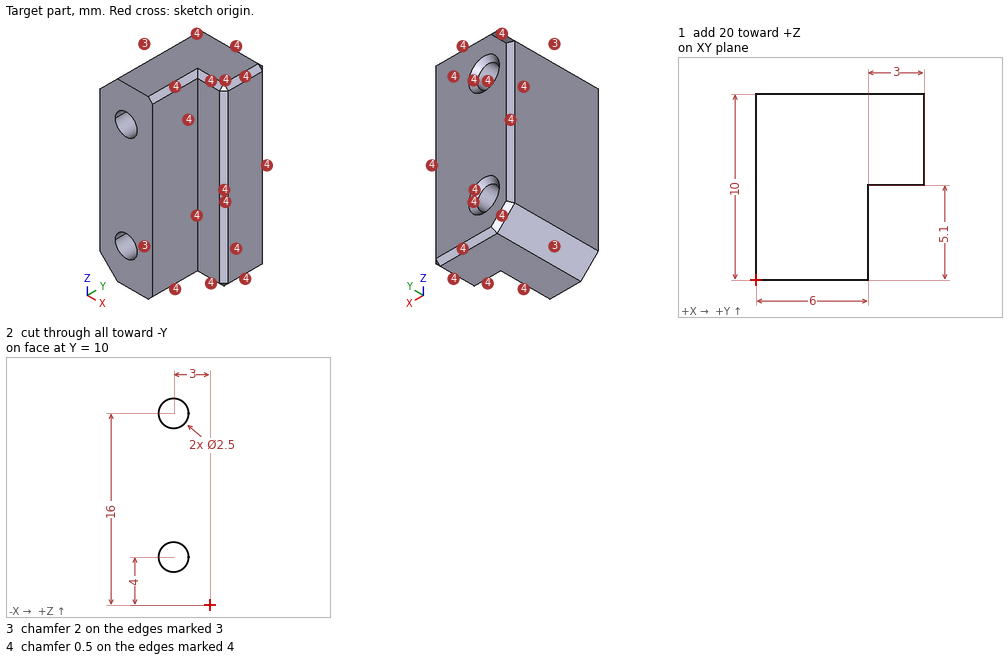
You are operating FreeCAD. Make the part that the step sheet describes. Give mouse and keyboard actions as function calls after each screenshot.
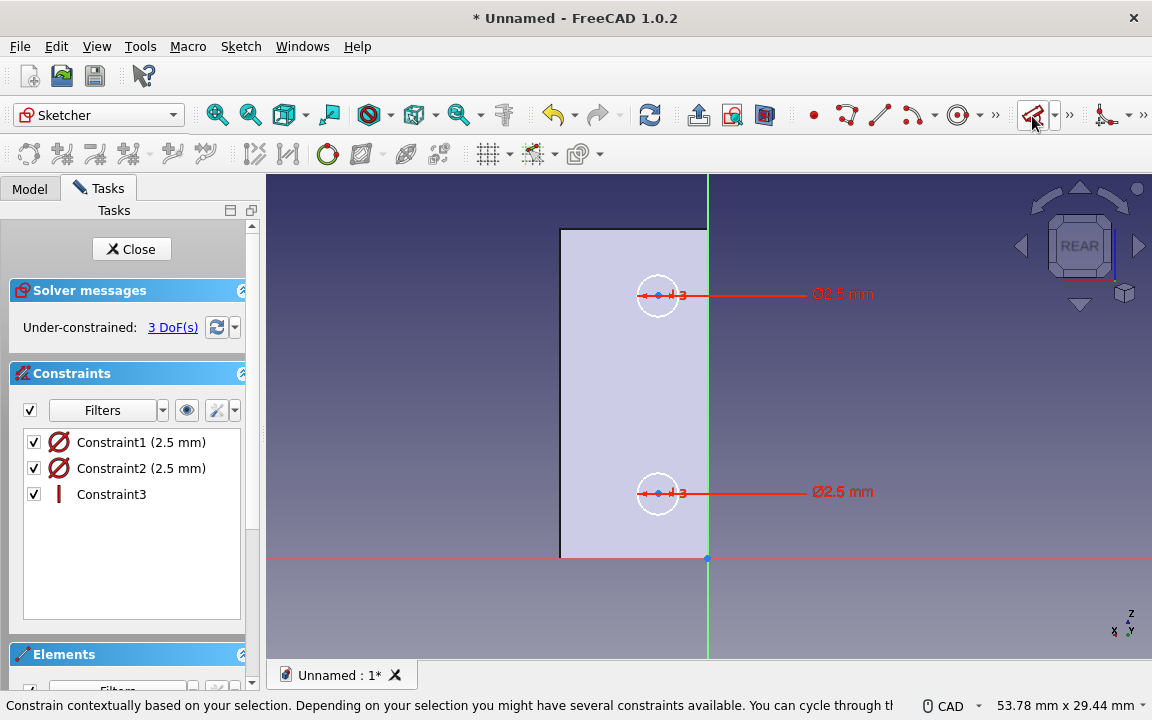
click(658, 296)
click(683, 593)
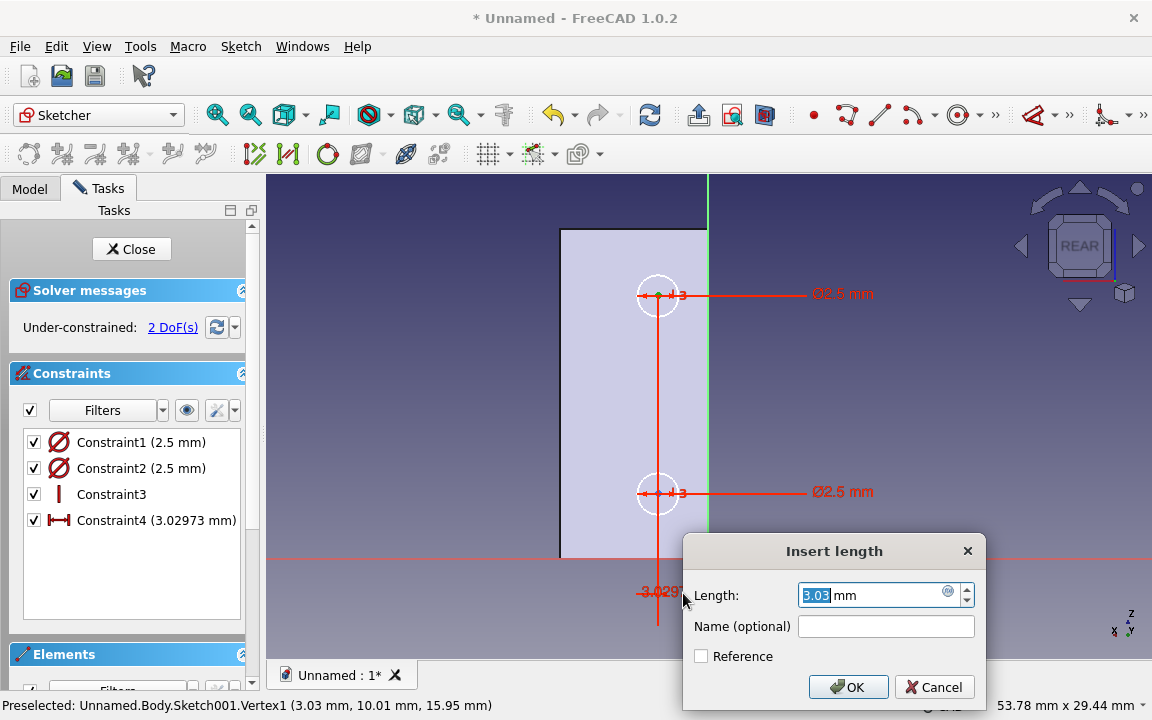
text(3)
key(Return)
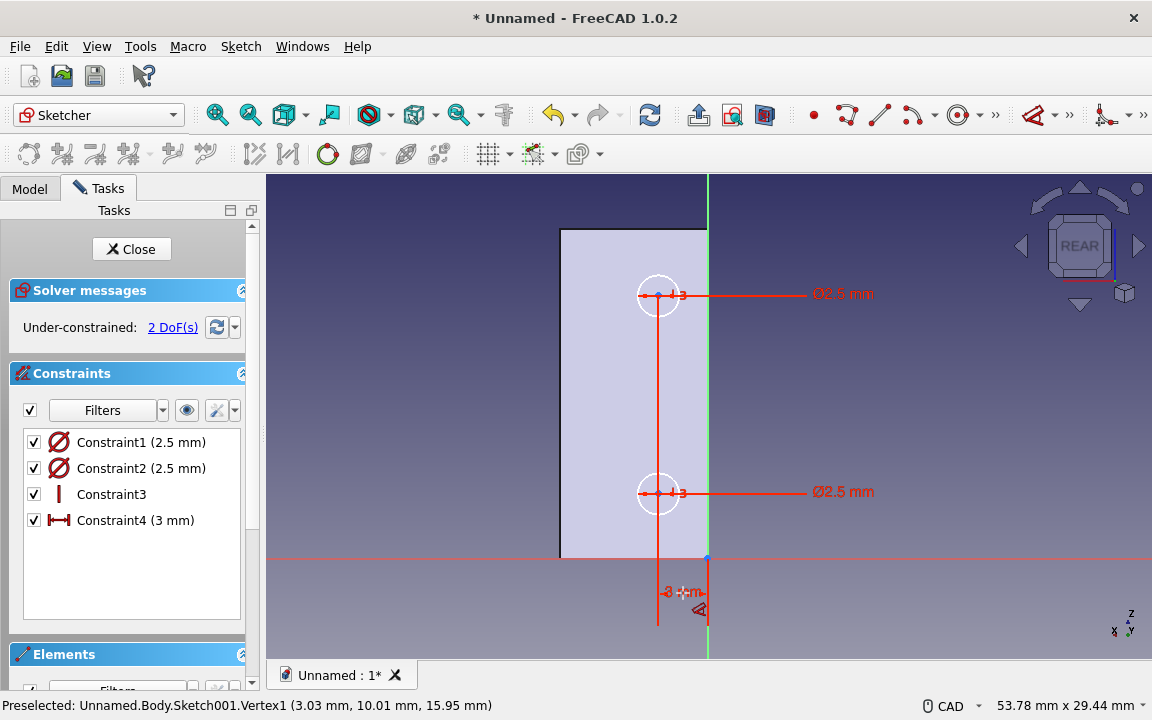
click(658, 494)
click(742, 526)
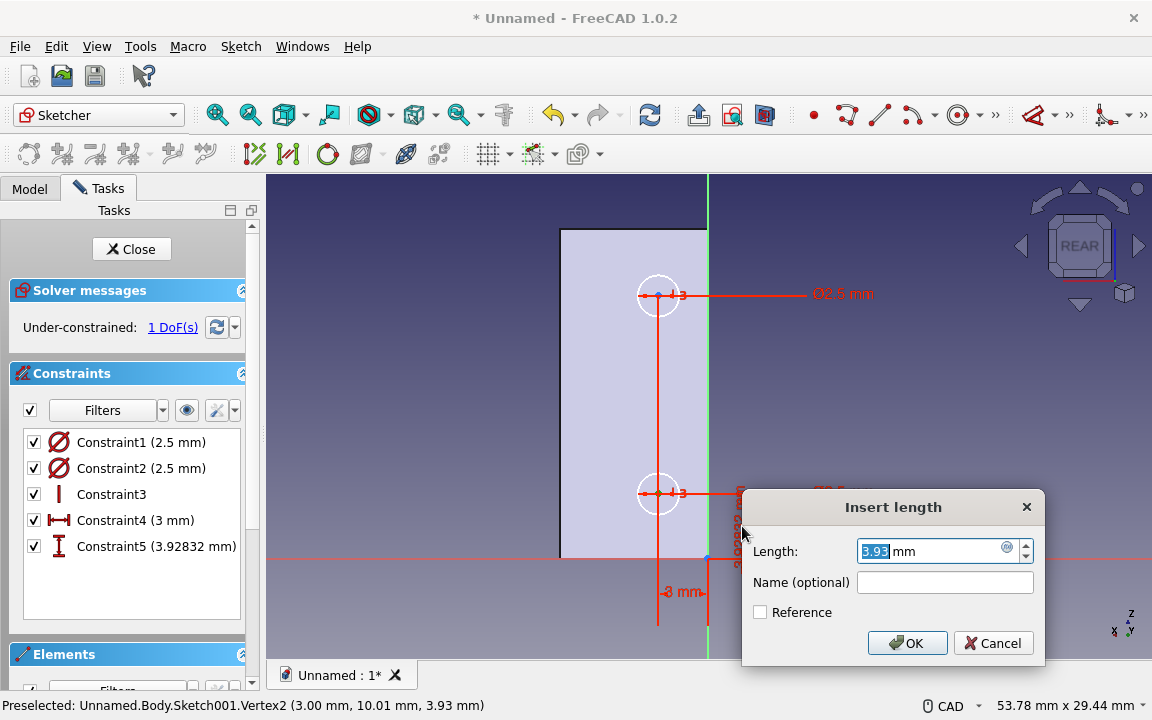
text(4)
key(Return)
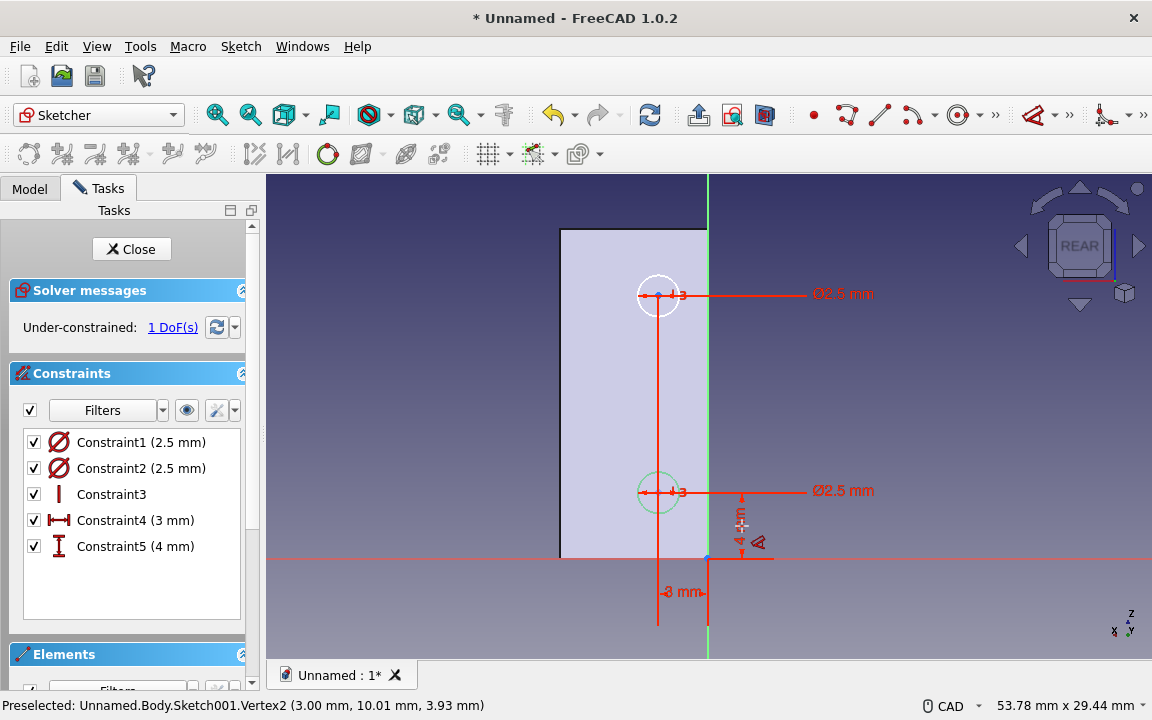
click(658, 296)
click(742, 427)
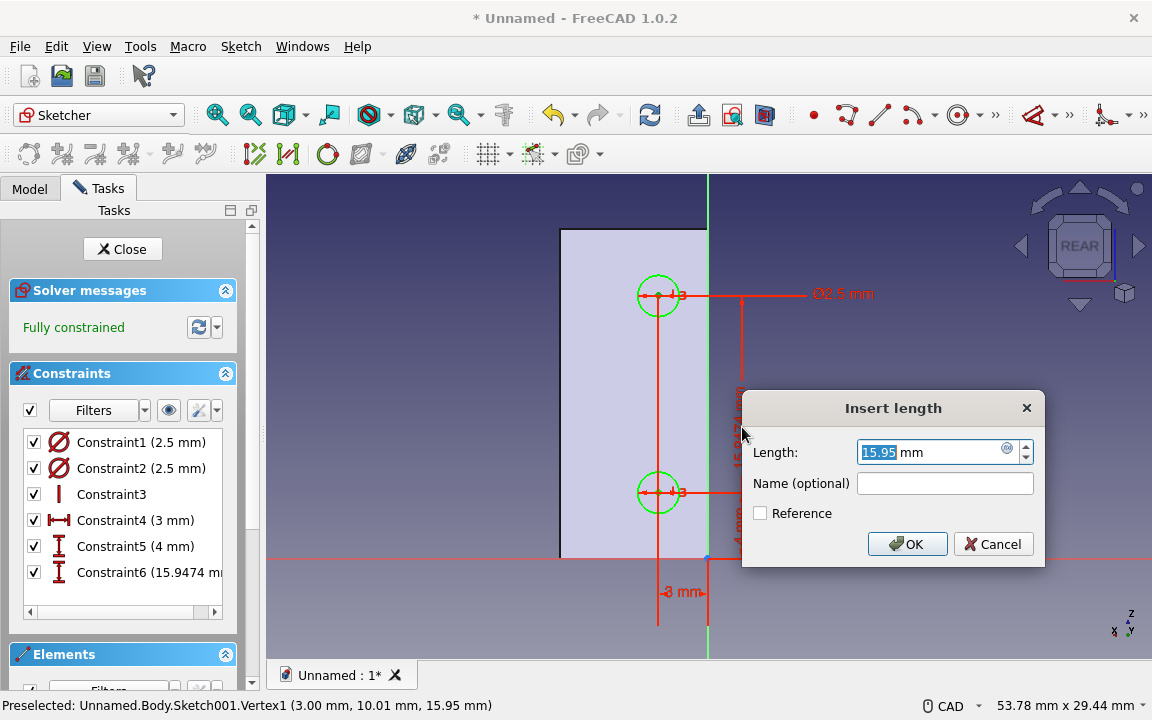
text(16)
key(Return)
key(Escape)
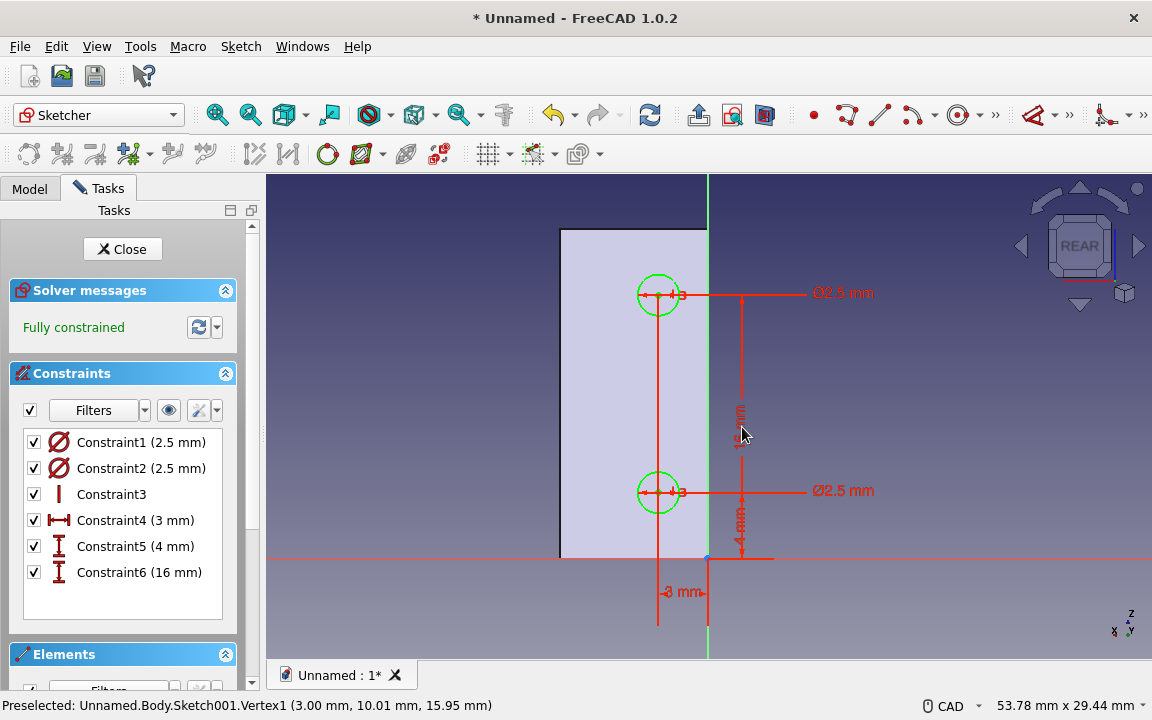
click(123, 249)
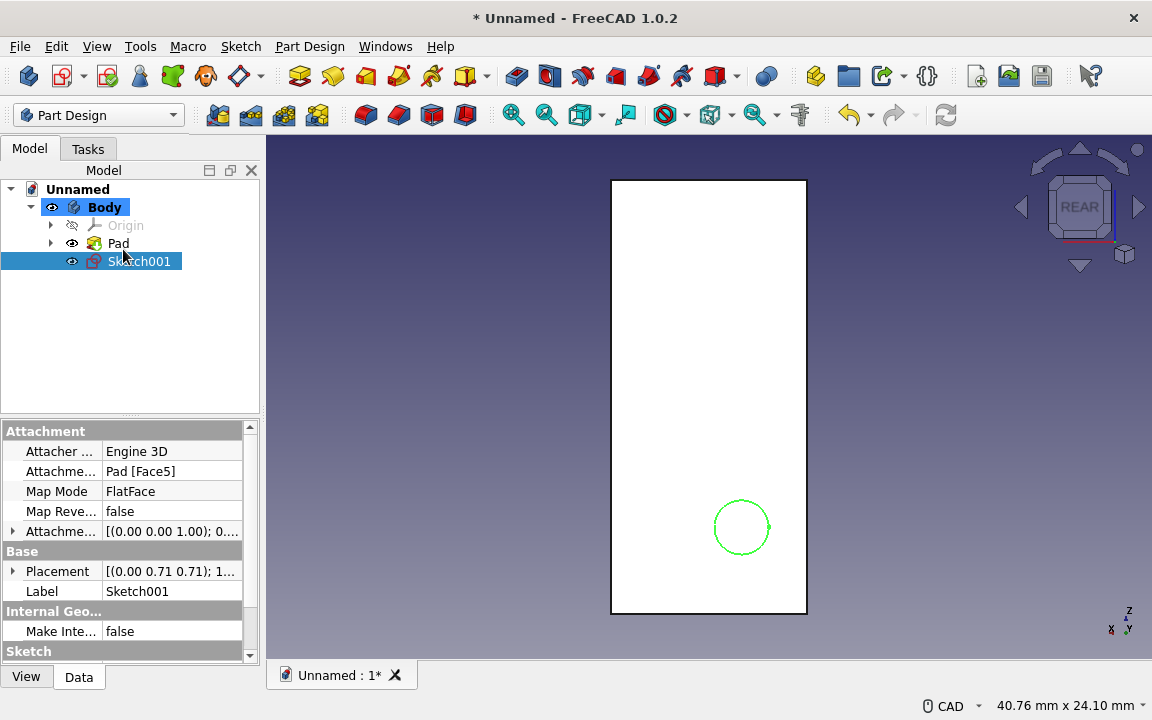
click(517, 76)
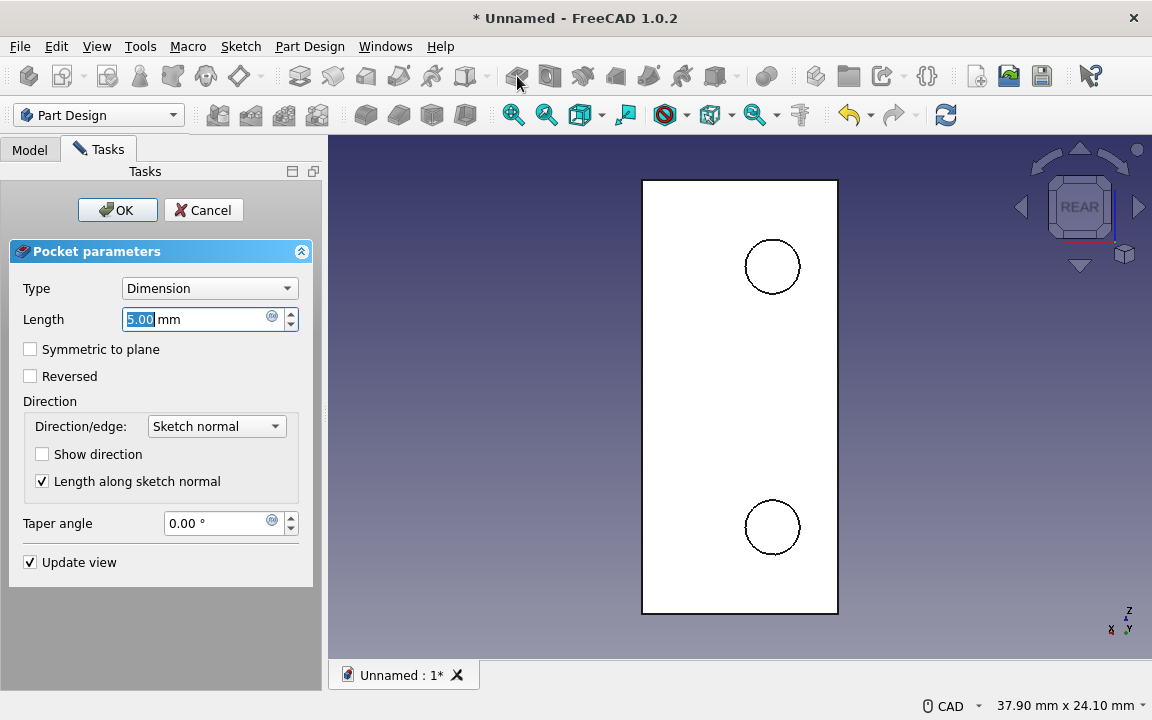
click(210, 288)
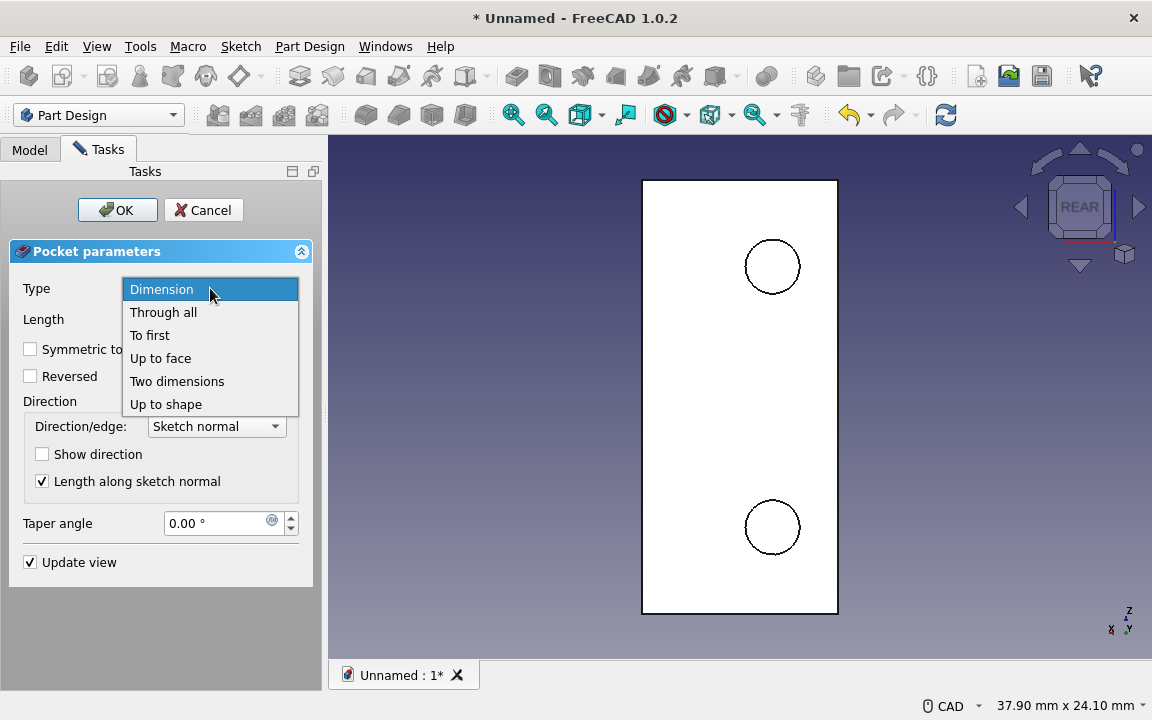
click(208, 312)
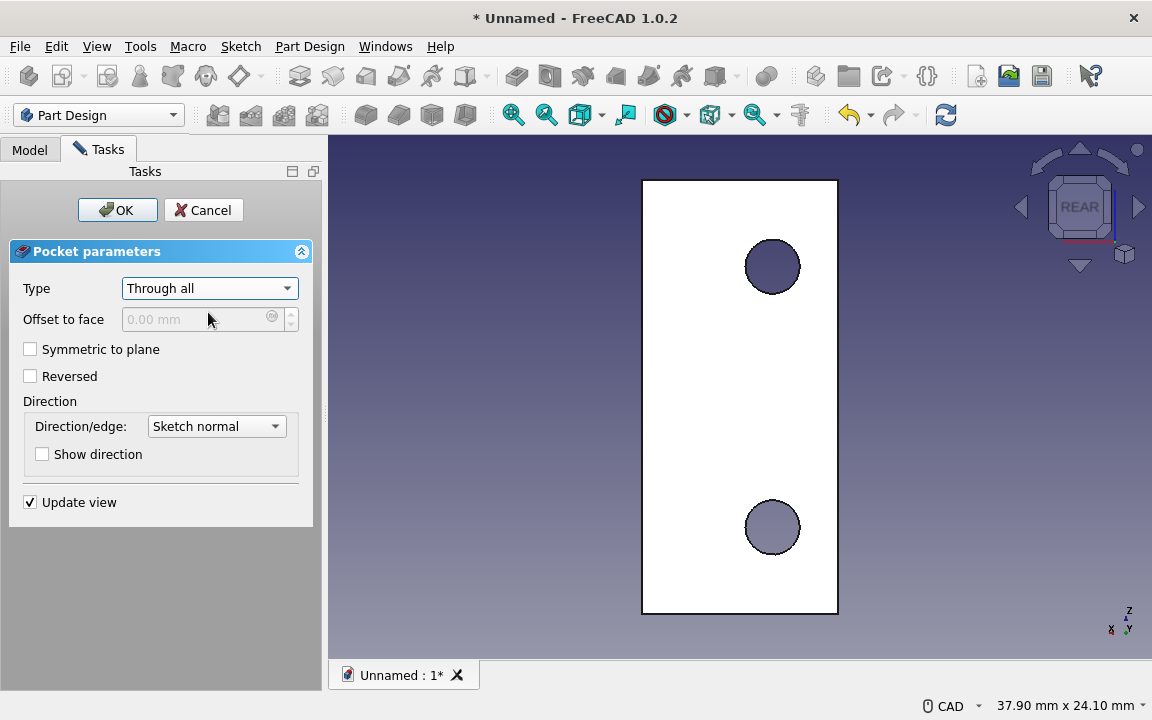
click(118, 210)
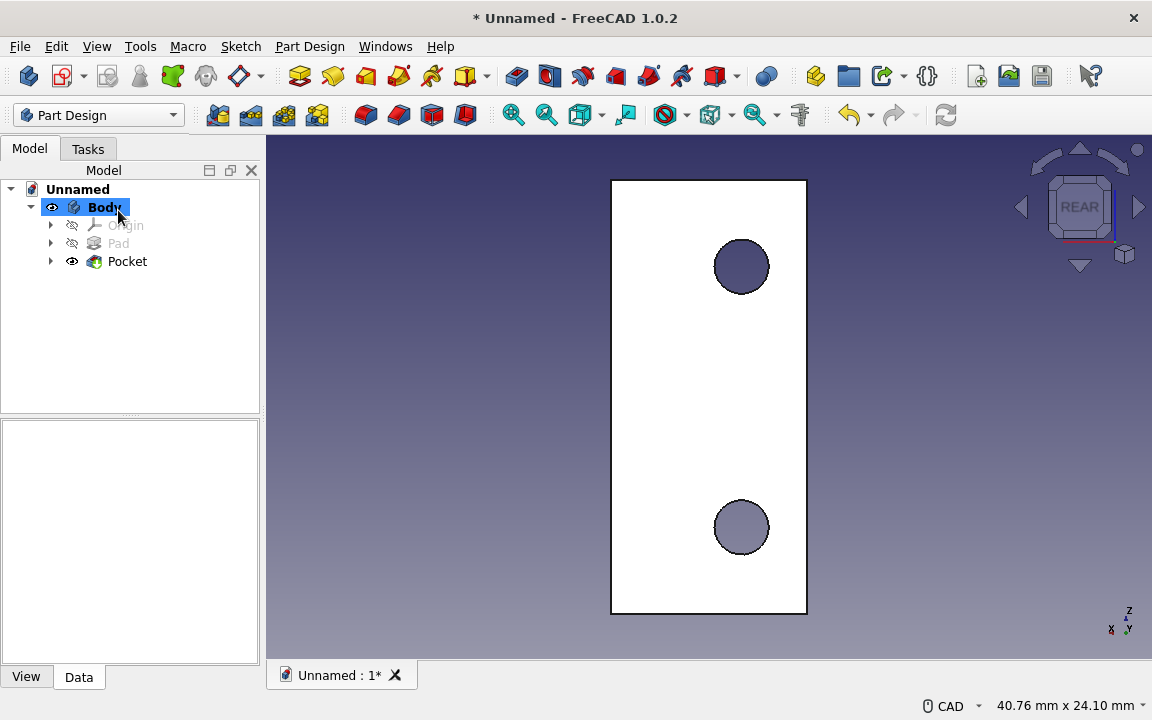
key(0)